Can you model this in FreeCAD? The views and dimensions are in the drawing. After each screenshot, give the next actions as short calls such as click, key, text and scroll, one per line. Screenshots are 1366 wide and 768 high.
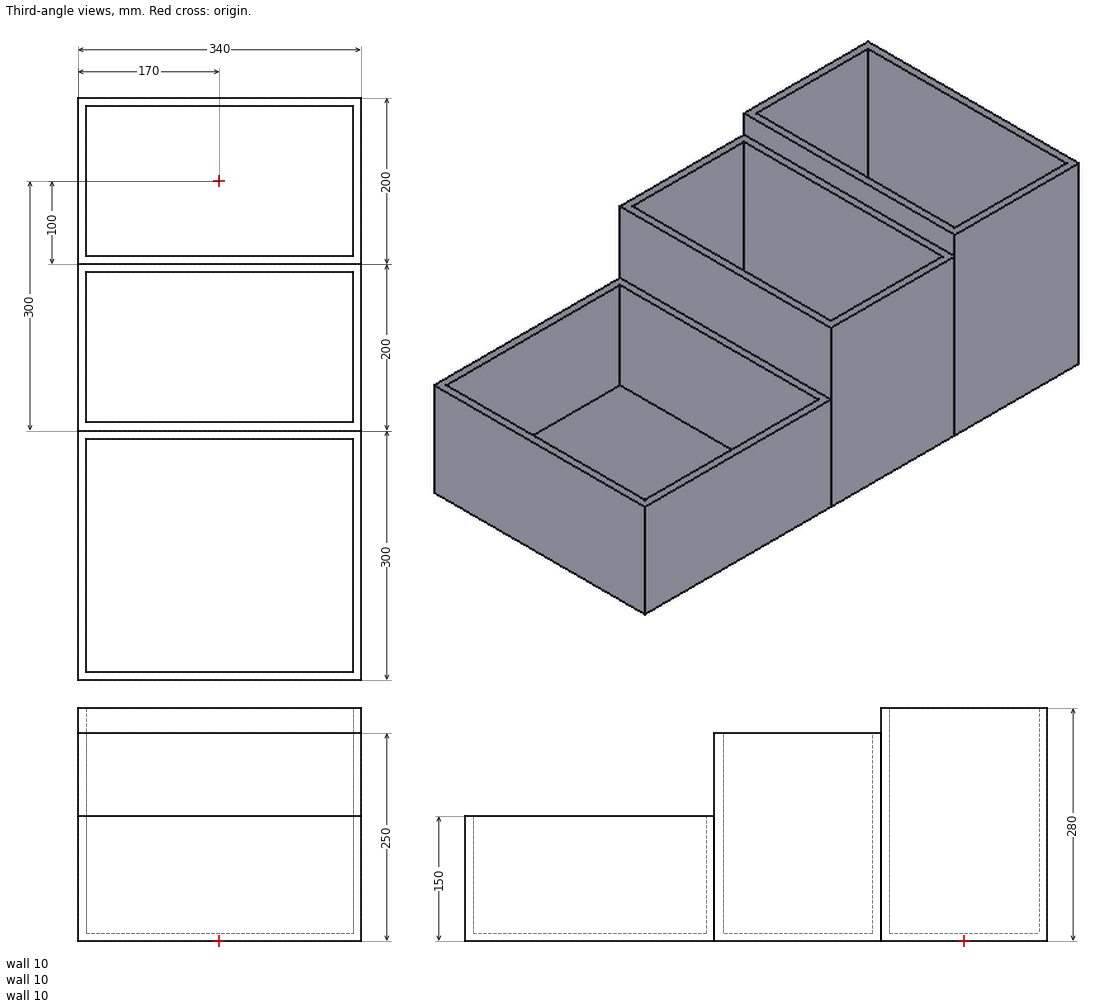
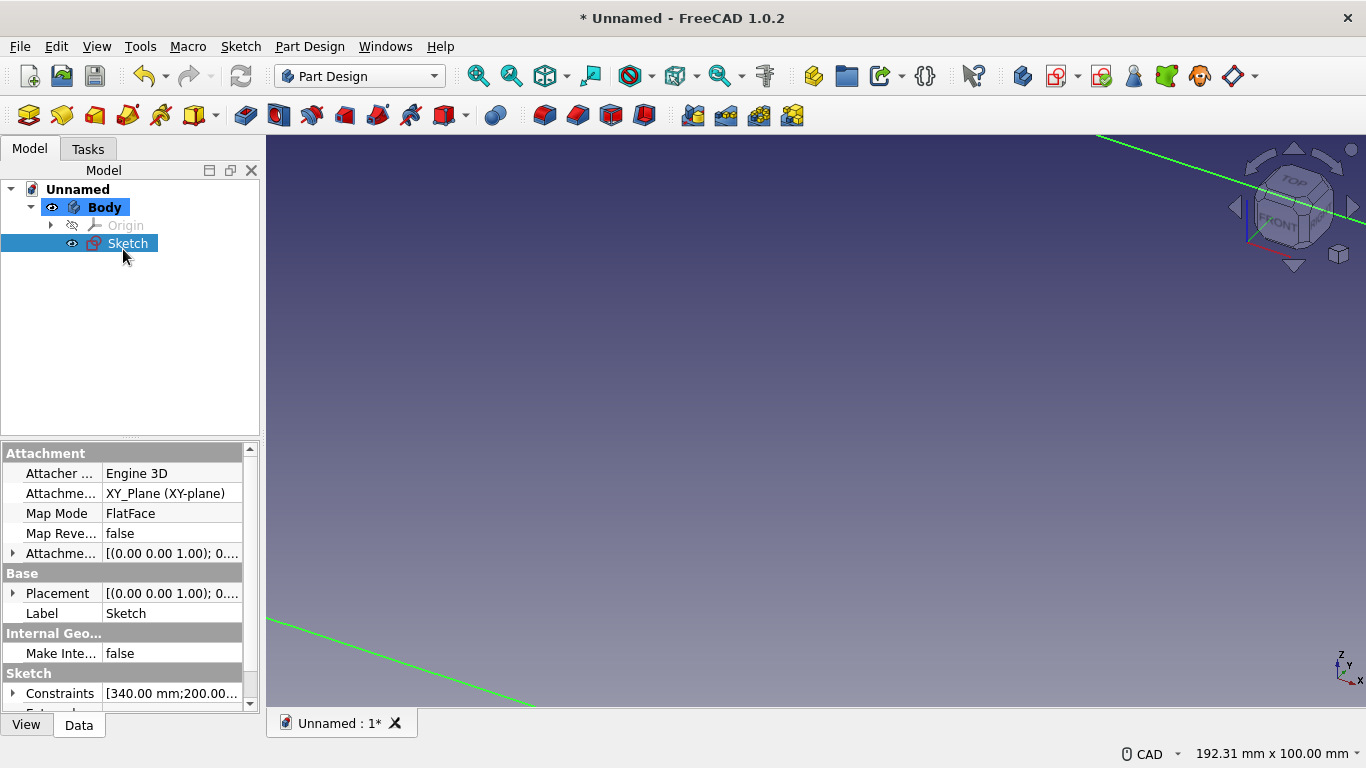
click(29, 116)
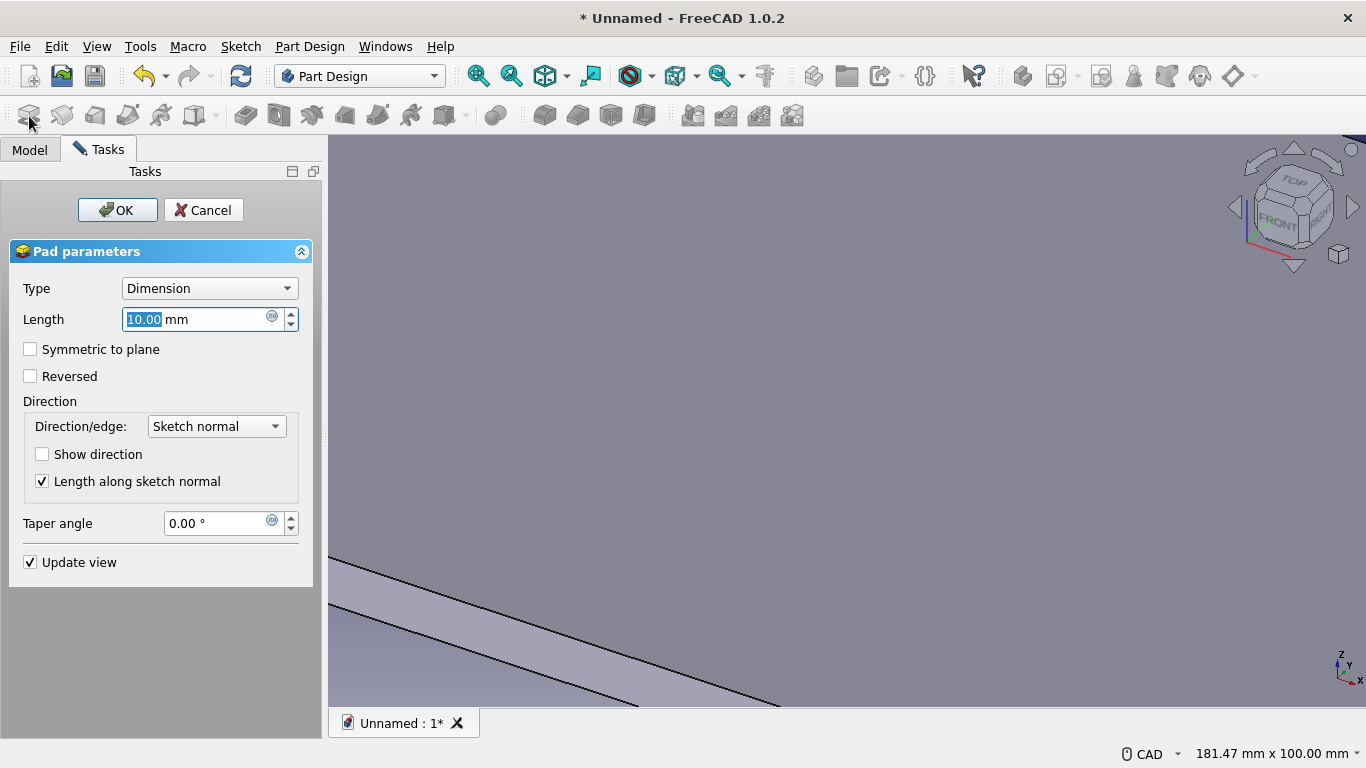
text(280)
key(Tab)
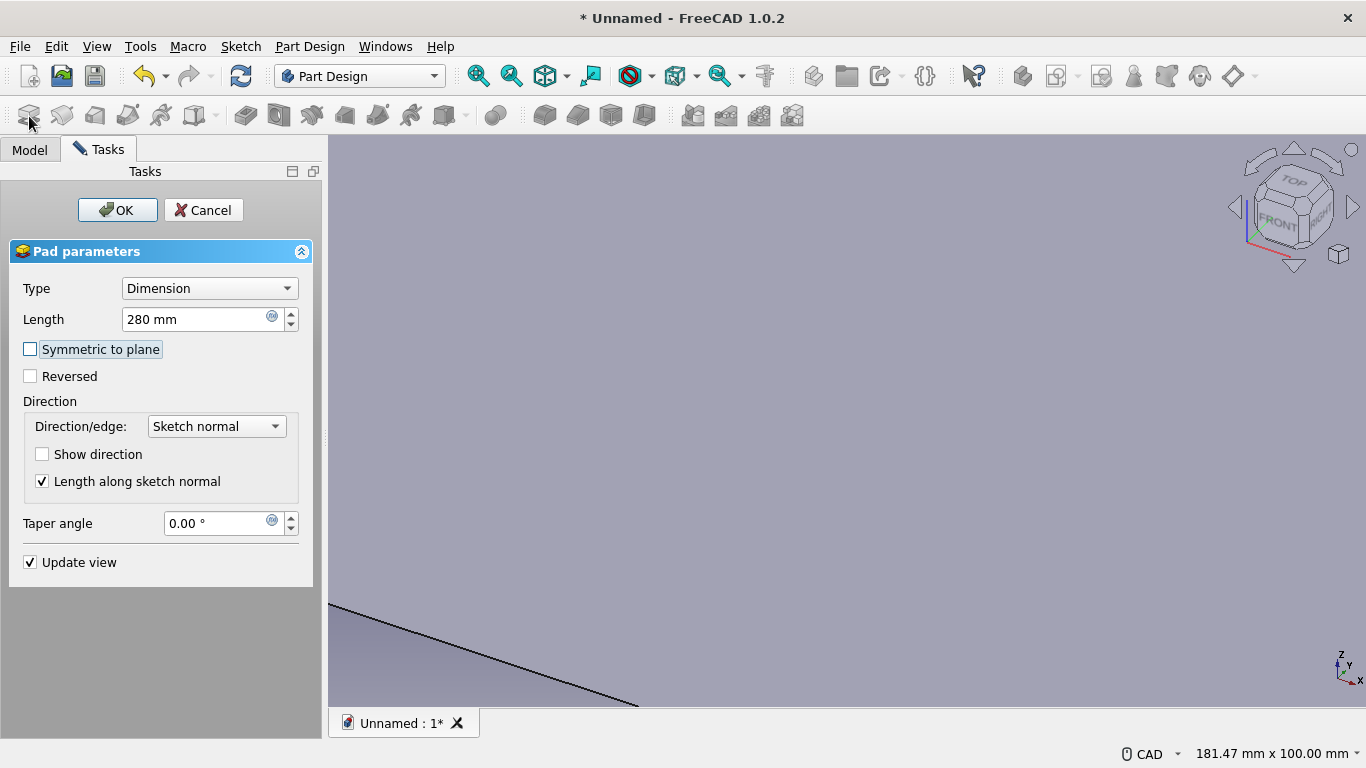
click(118, 210)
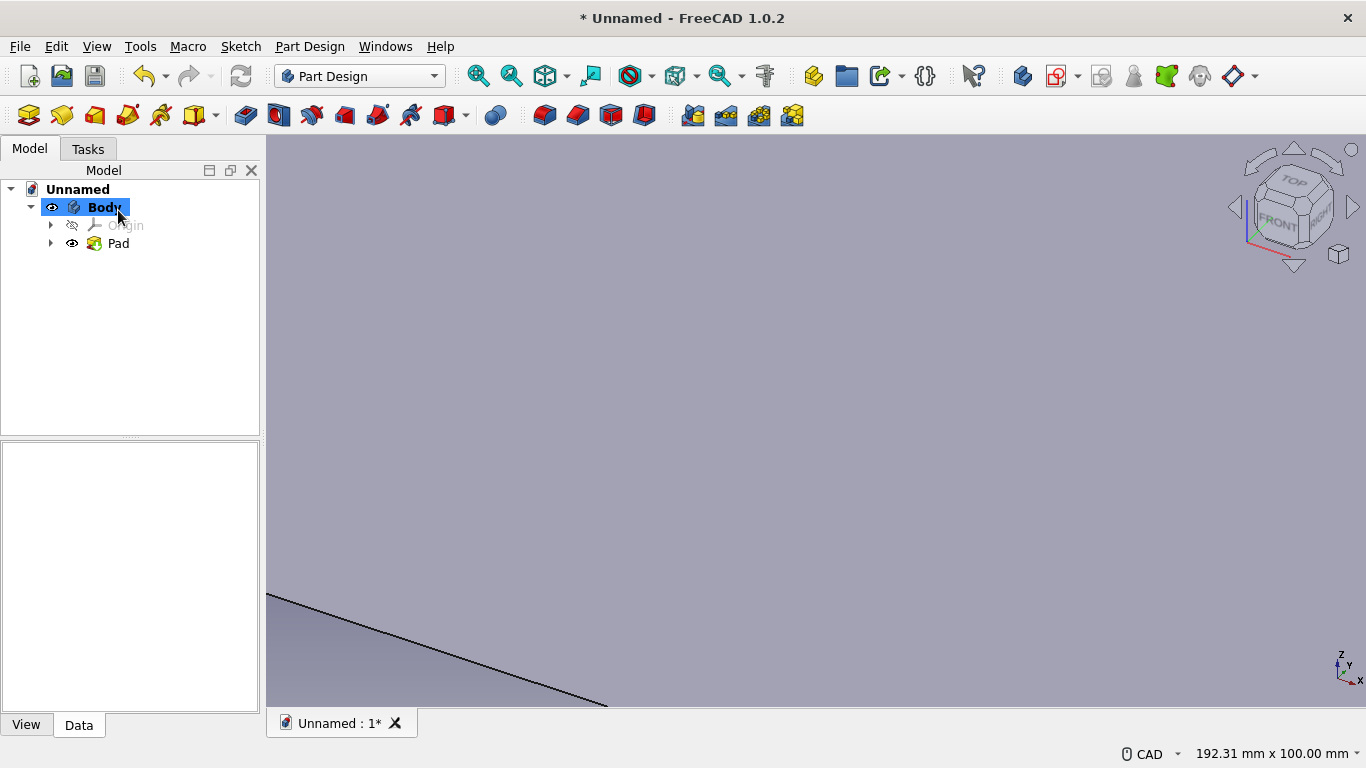
key(v)
key(f)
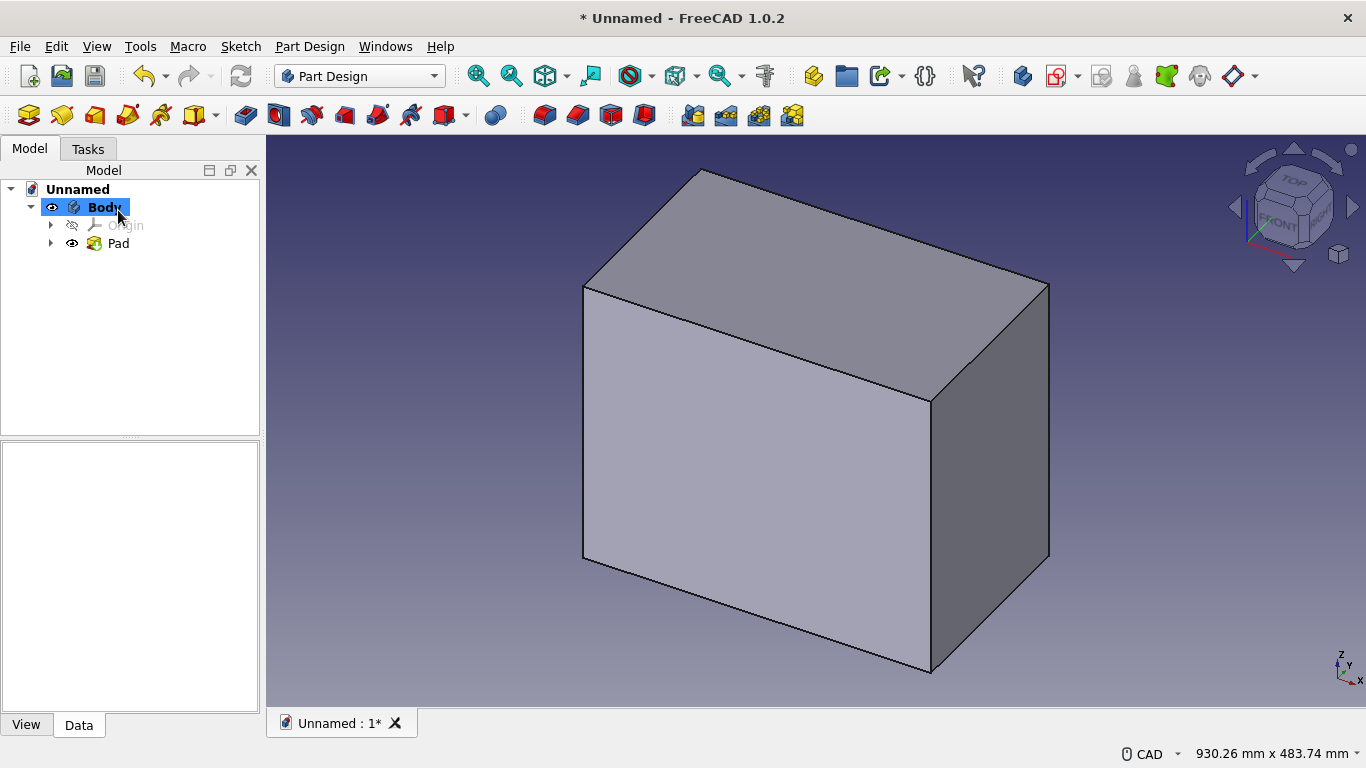
click(866, 301)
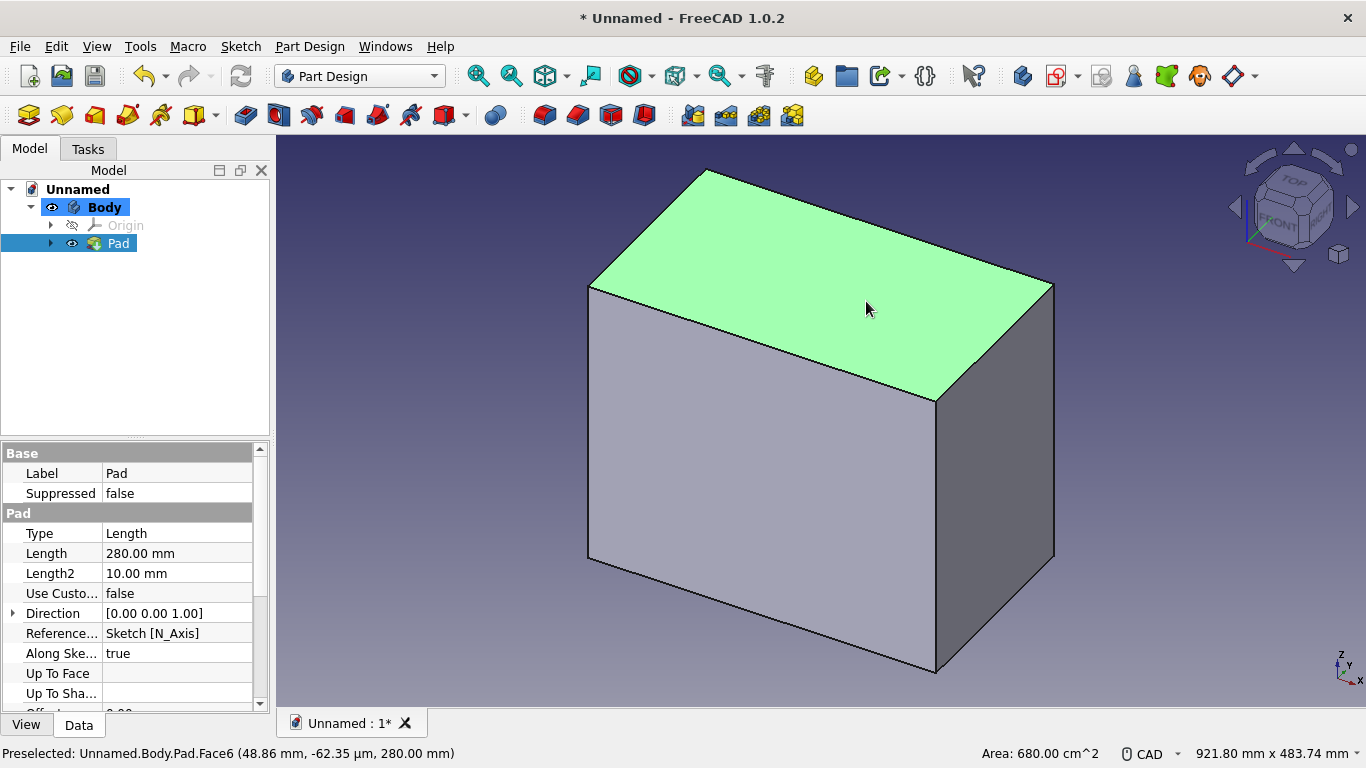
click(644, 116)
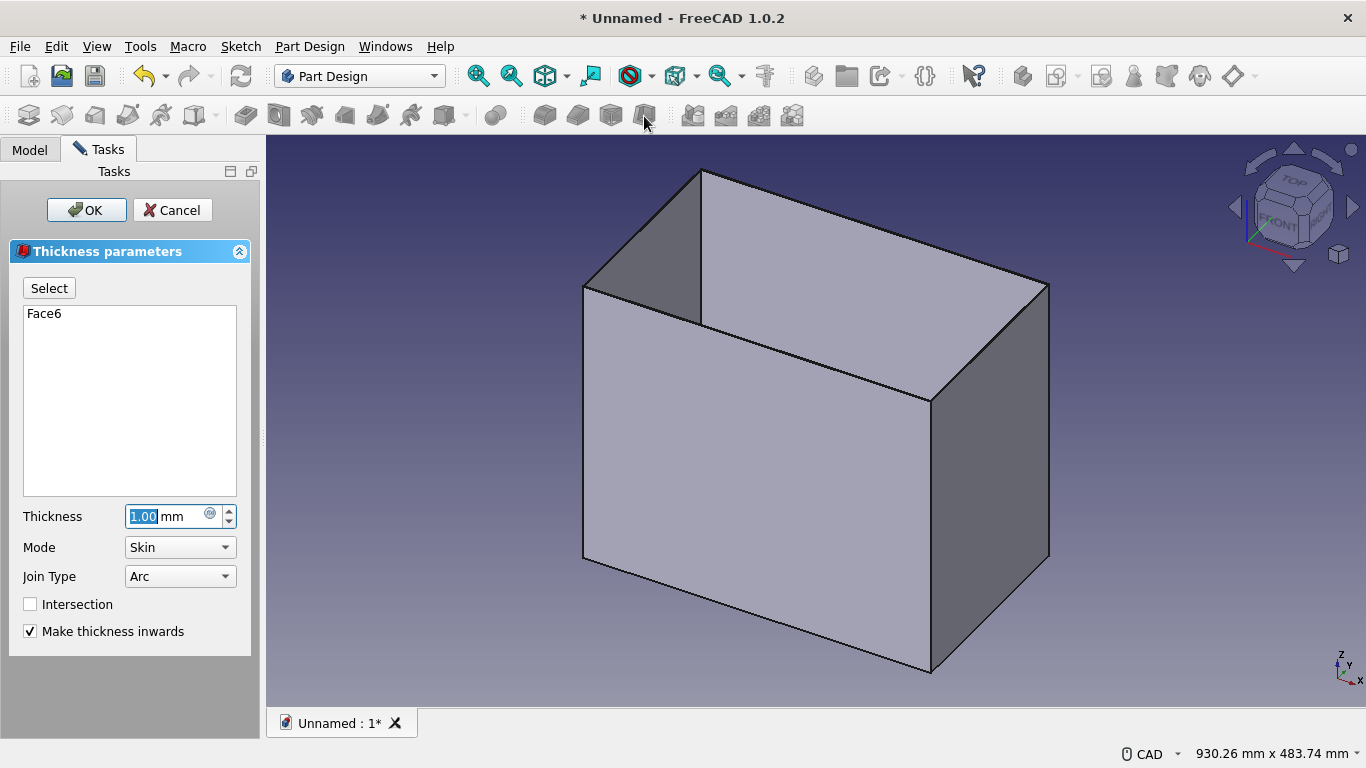
text(10)
key(Tab)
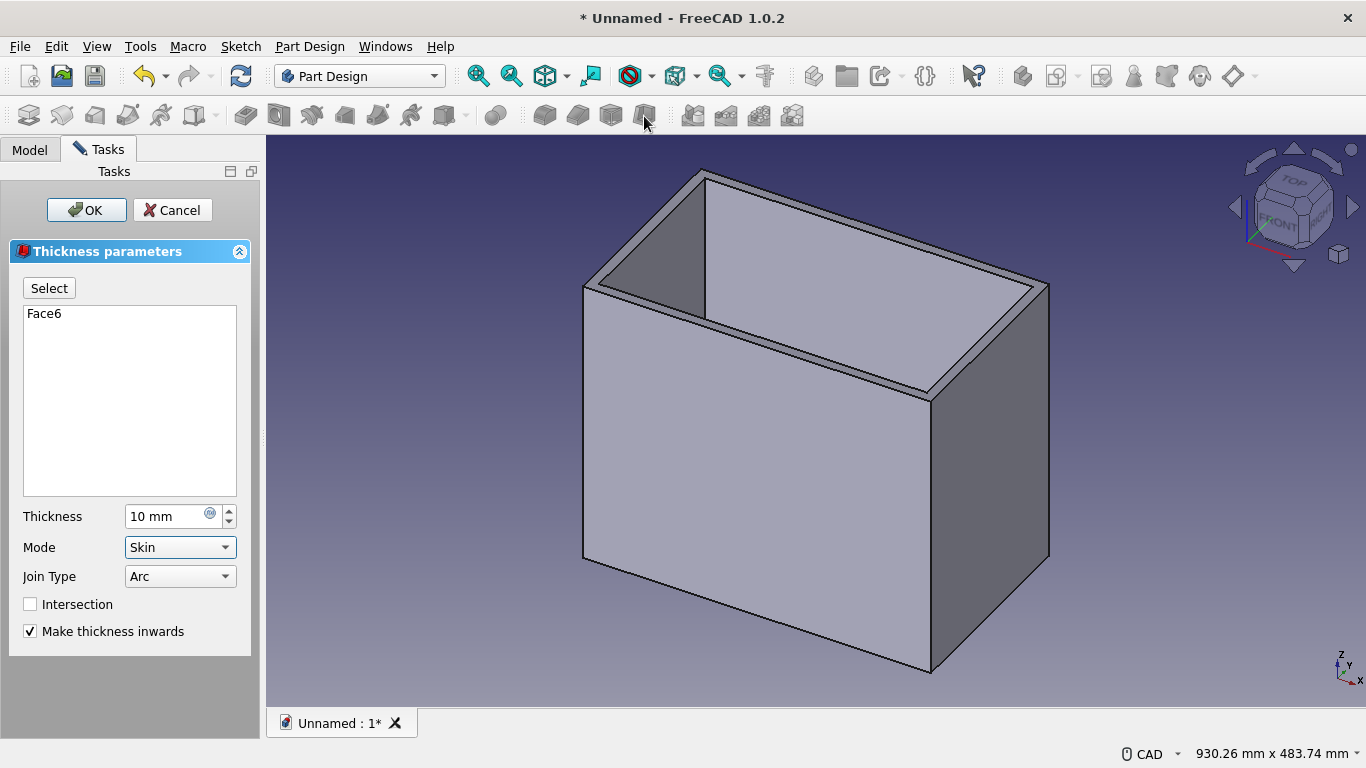
click(181, 576)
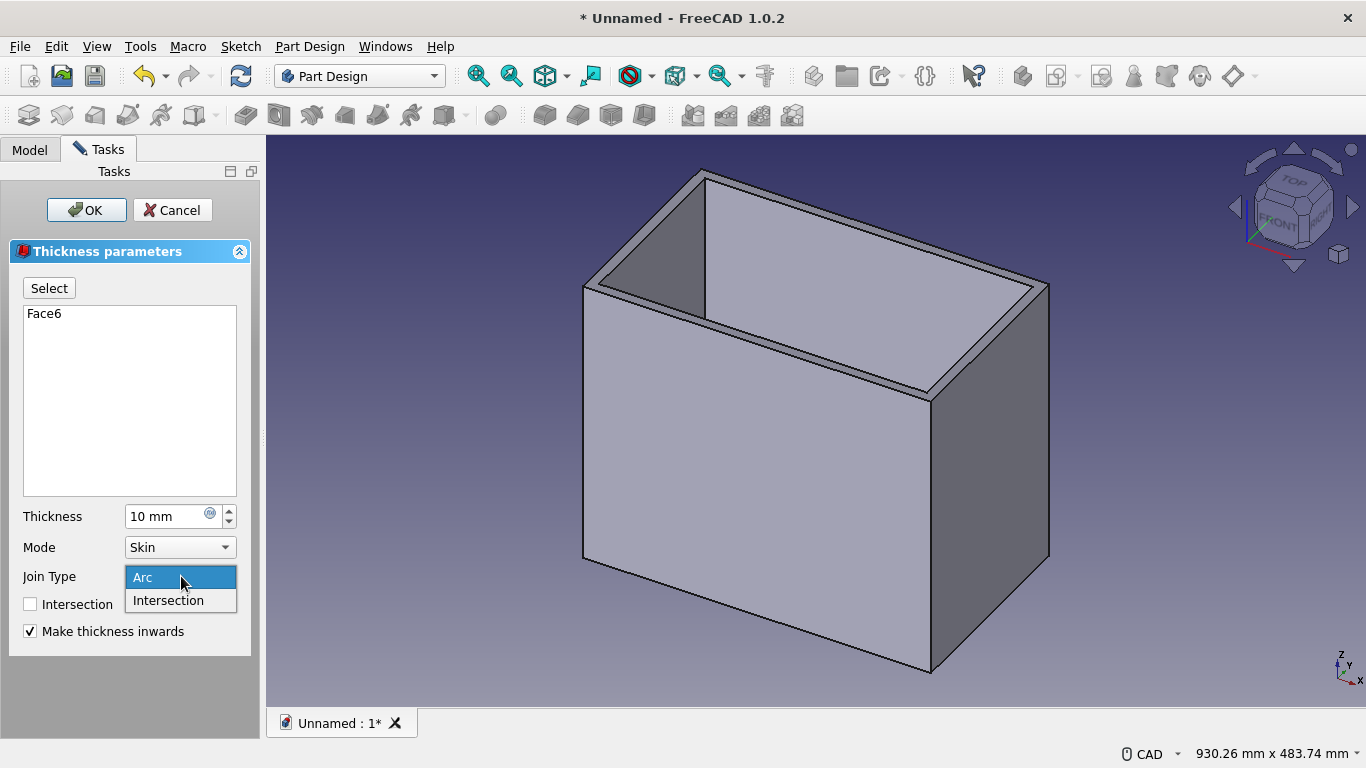
click(179, 600)